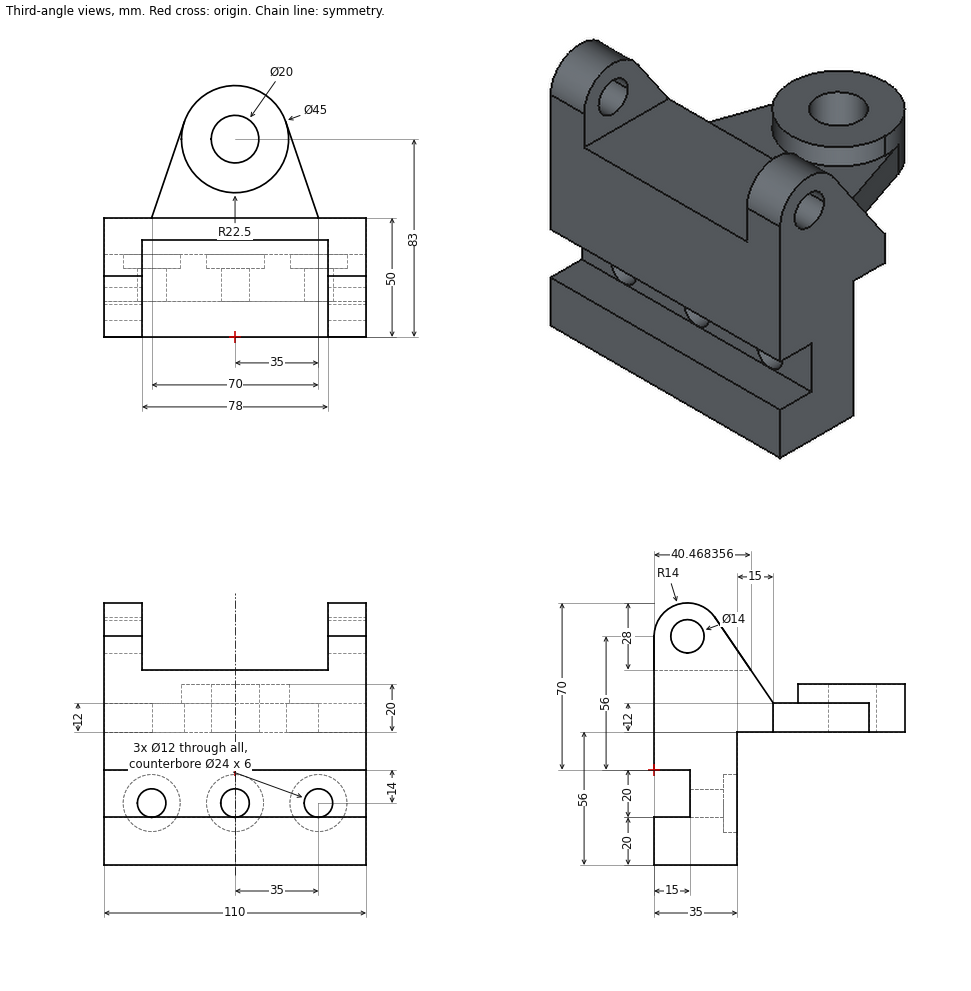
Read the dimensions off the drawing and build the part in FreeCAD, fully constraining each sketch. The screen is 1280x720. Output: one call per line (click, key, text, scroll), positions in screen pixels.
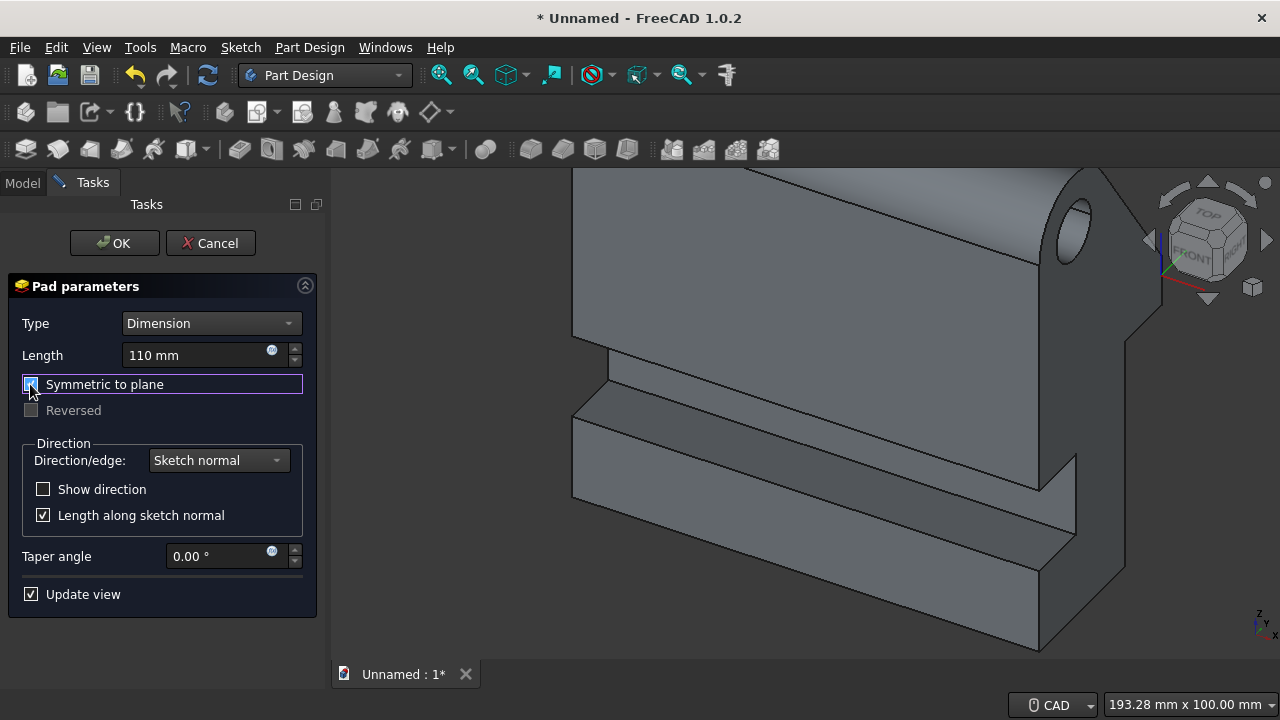
click(115, 243)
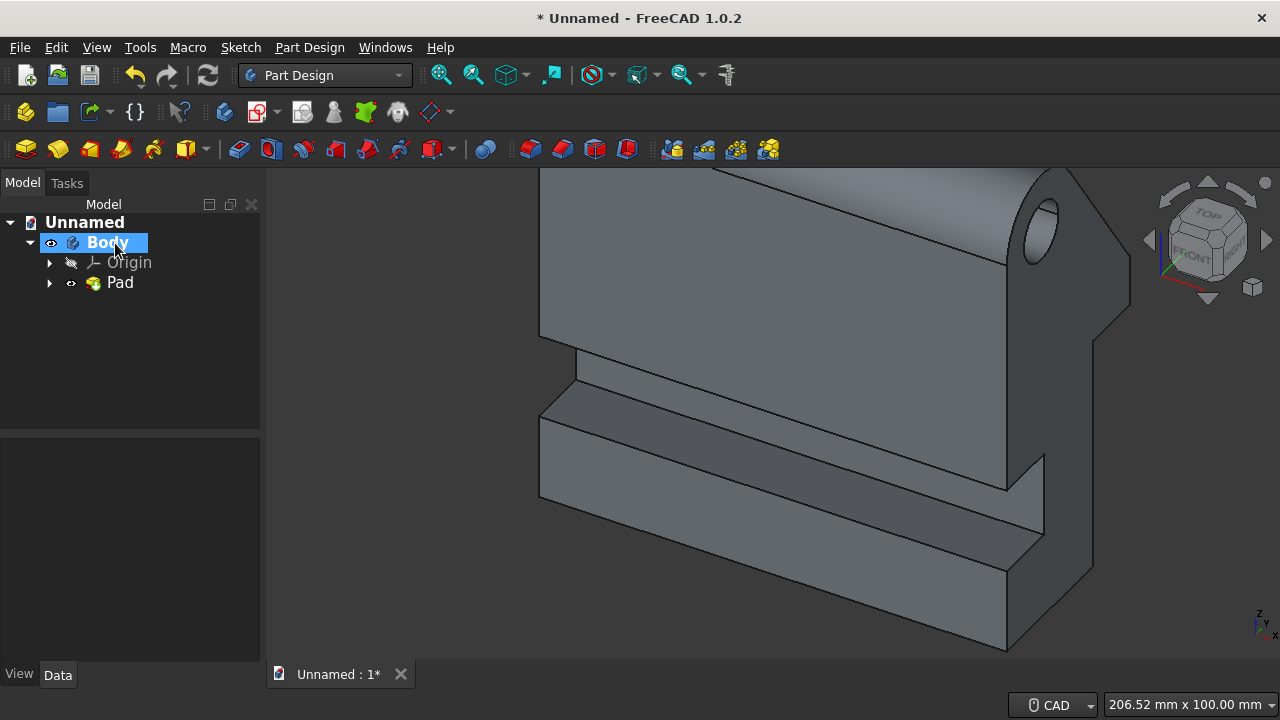
click(442, 76)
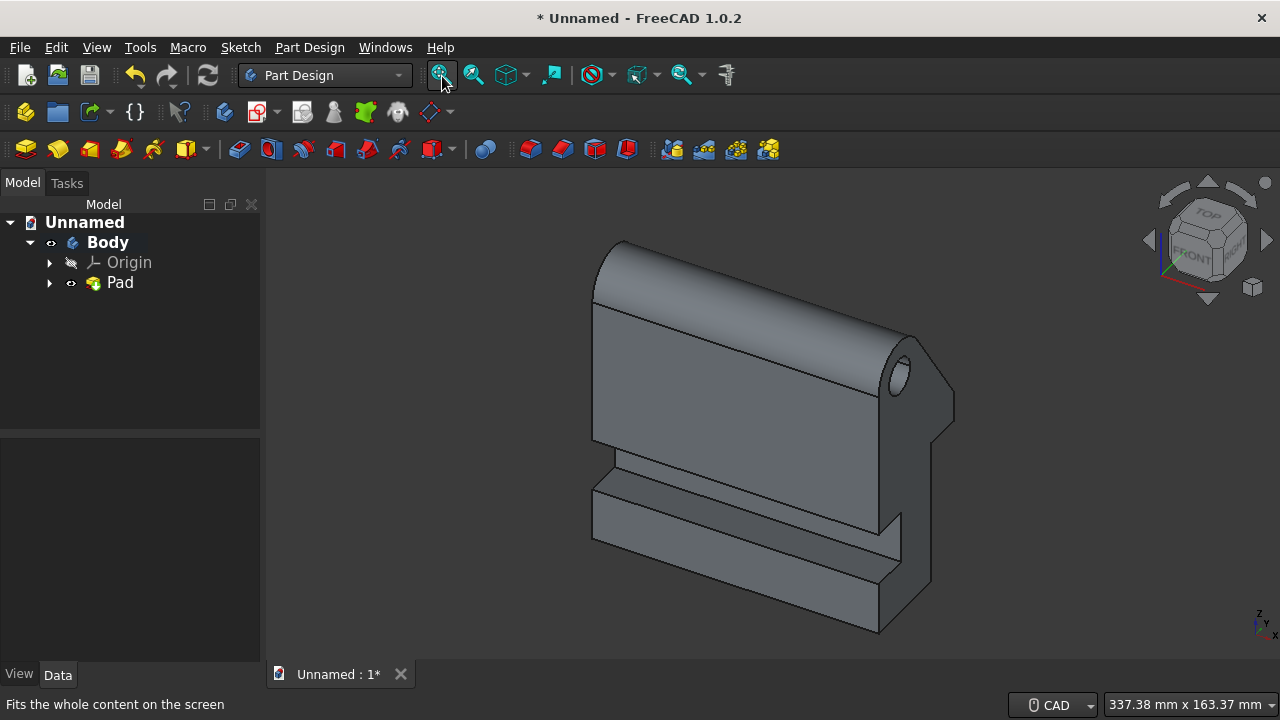
click(258, 112)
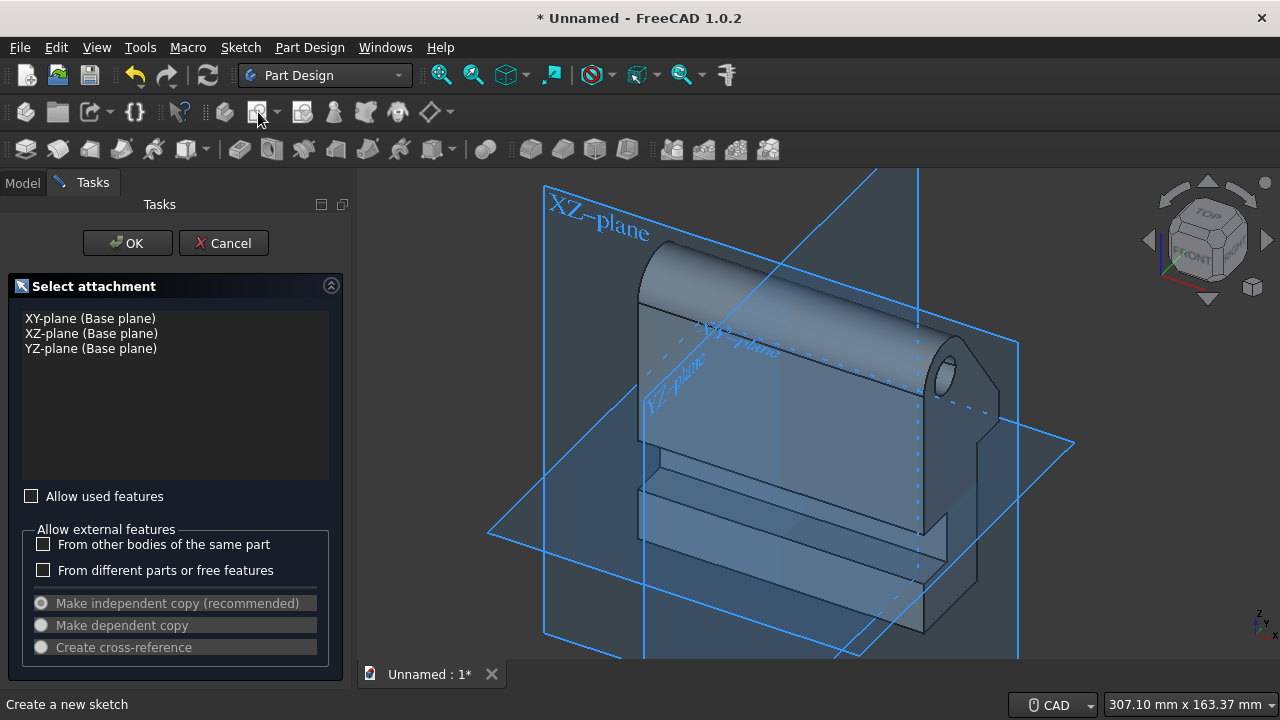
click(82, 348)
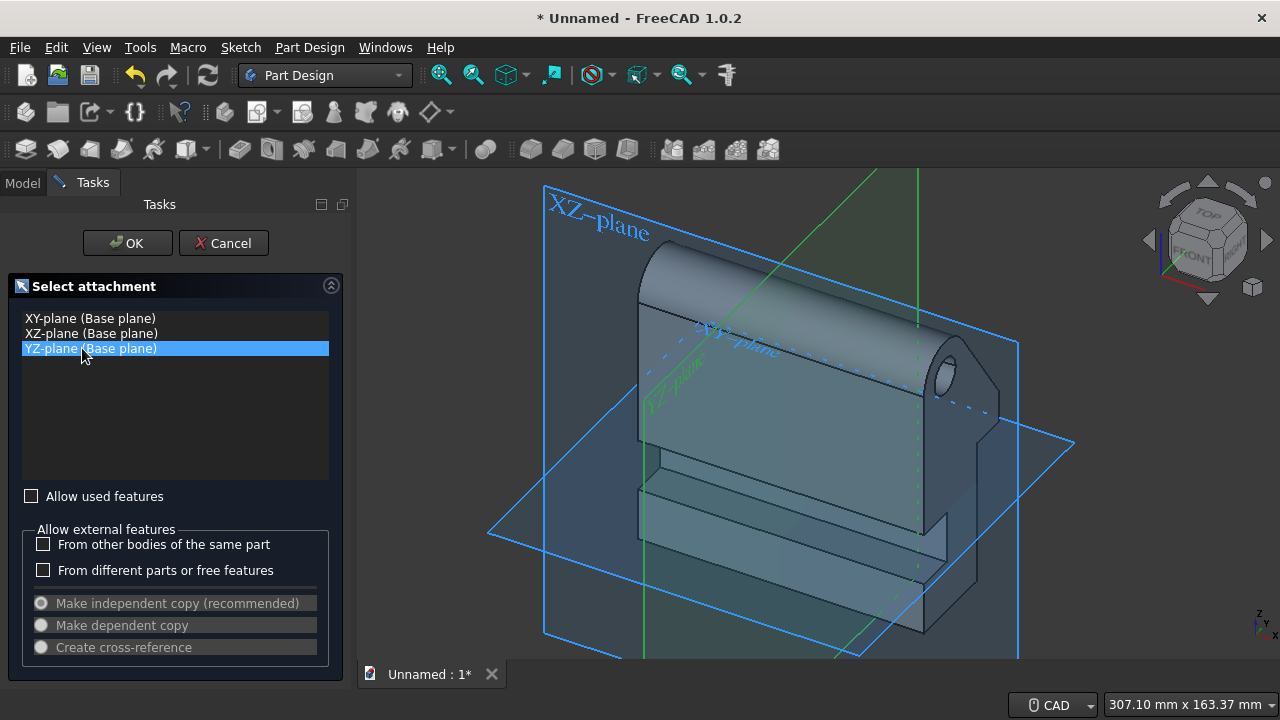
click(128, 243)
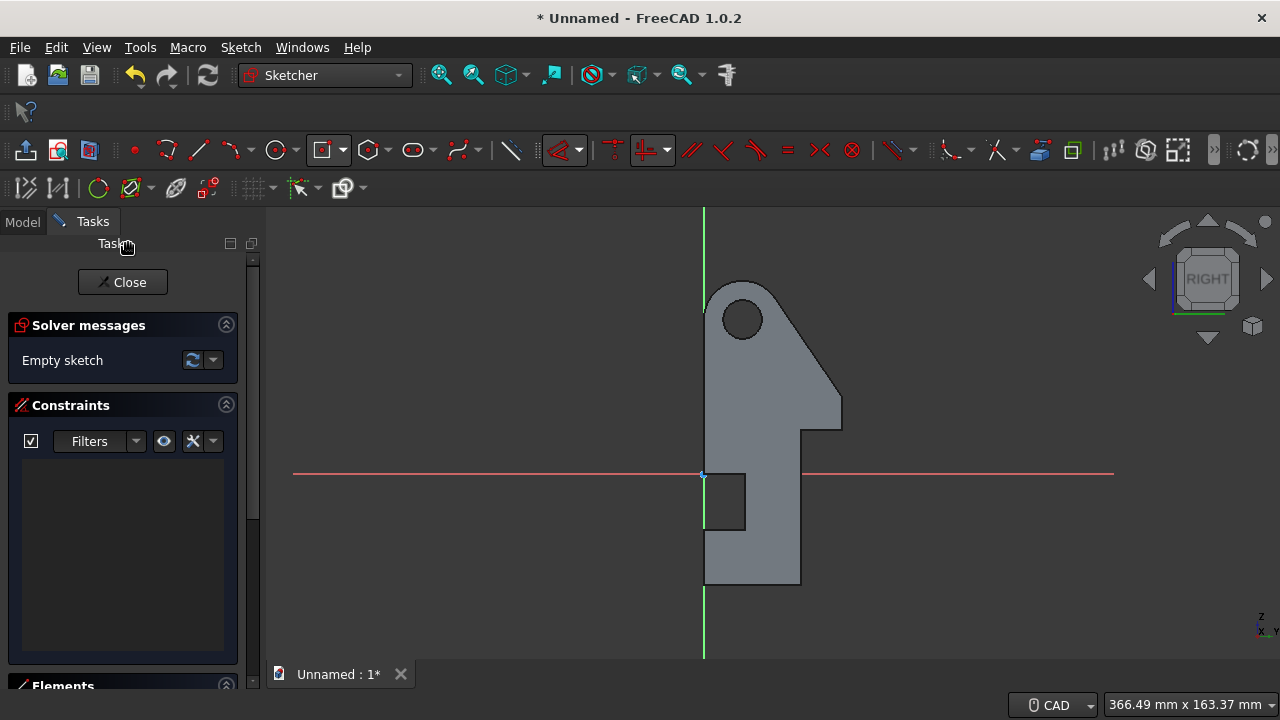
click(90, 150)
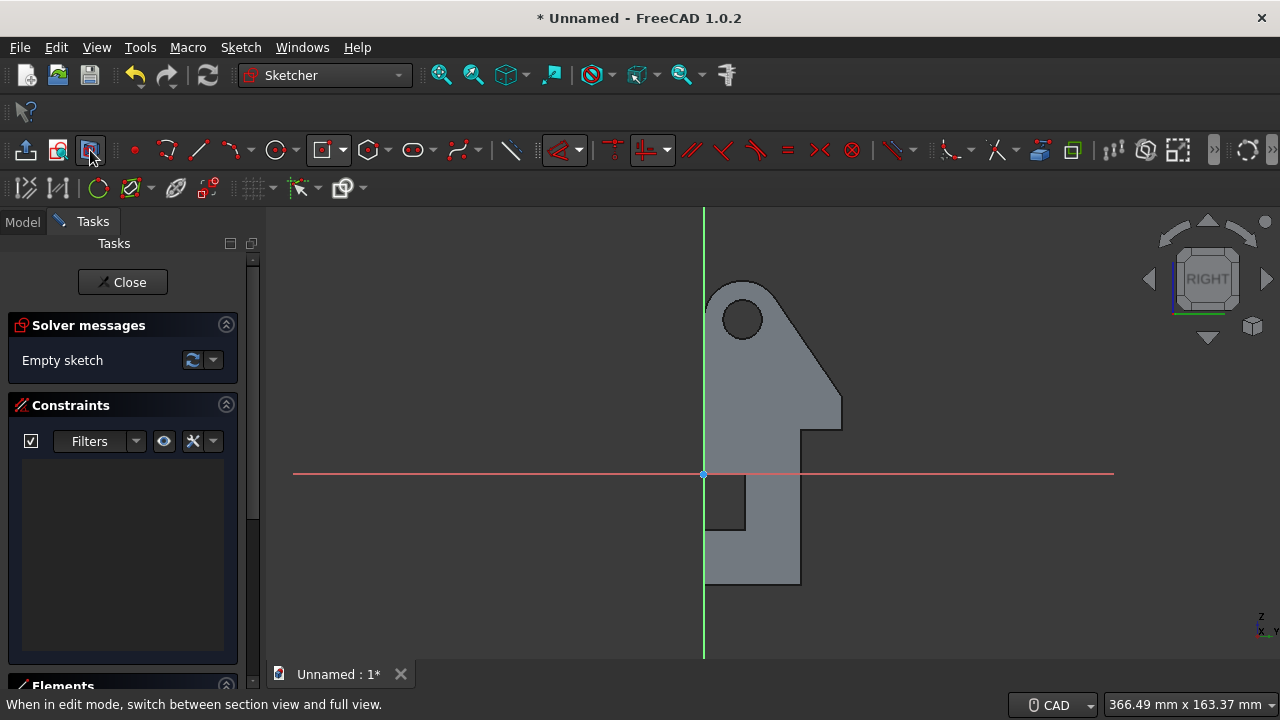
scroll(872, 265, up, 2)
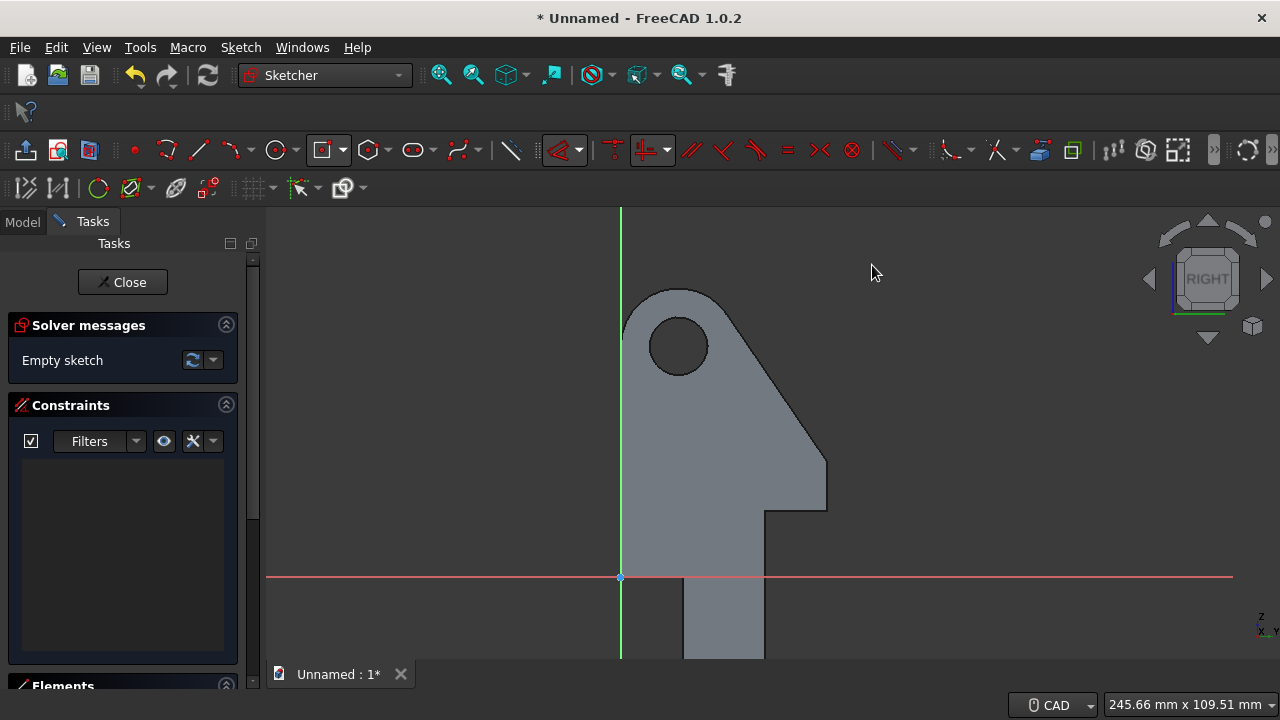
key(g)
key(r)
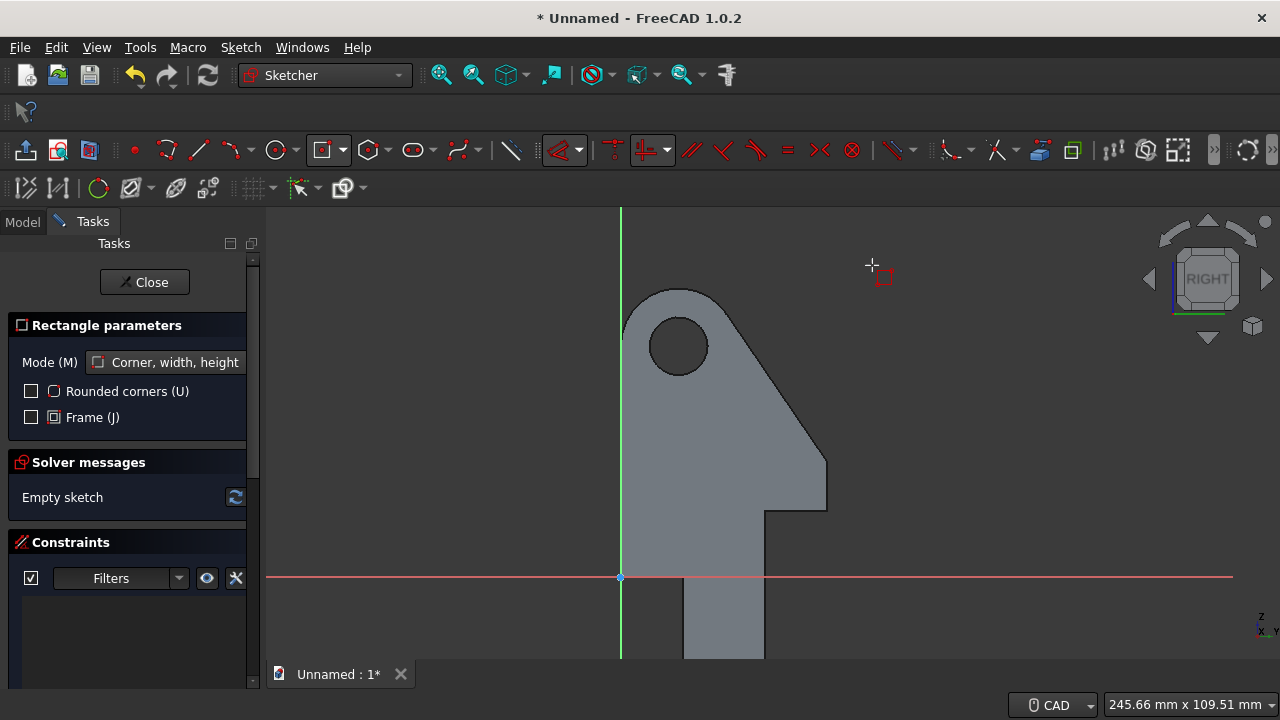
click(621, 288)
click(788, 404)
key(Escape)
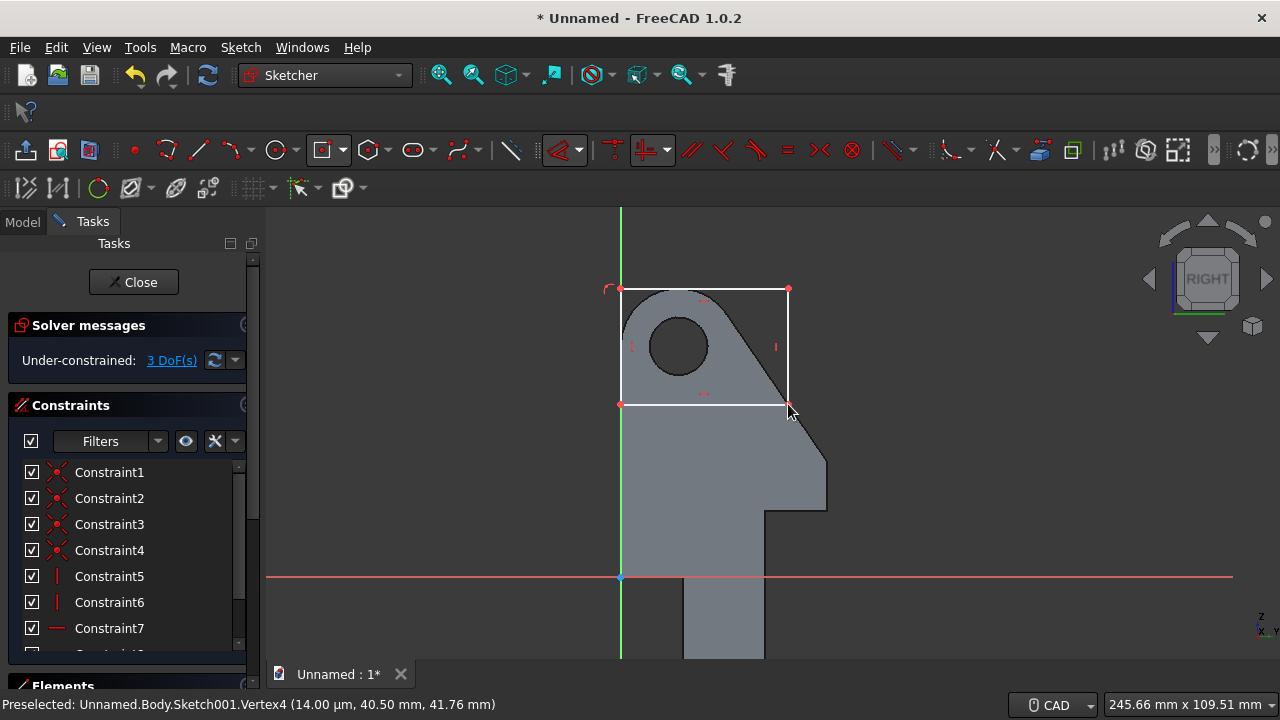
click(621, 324)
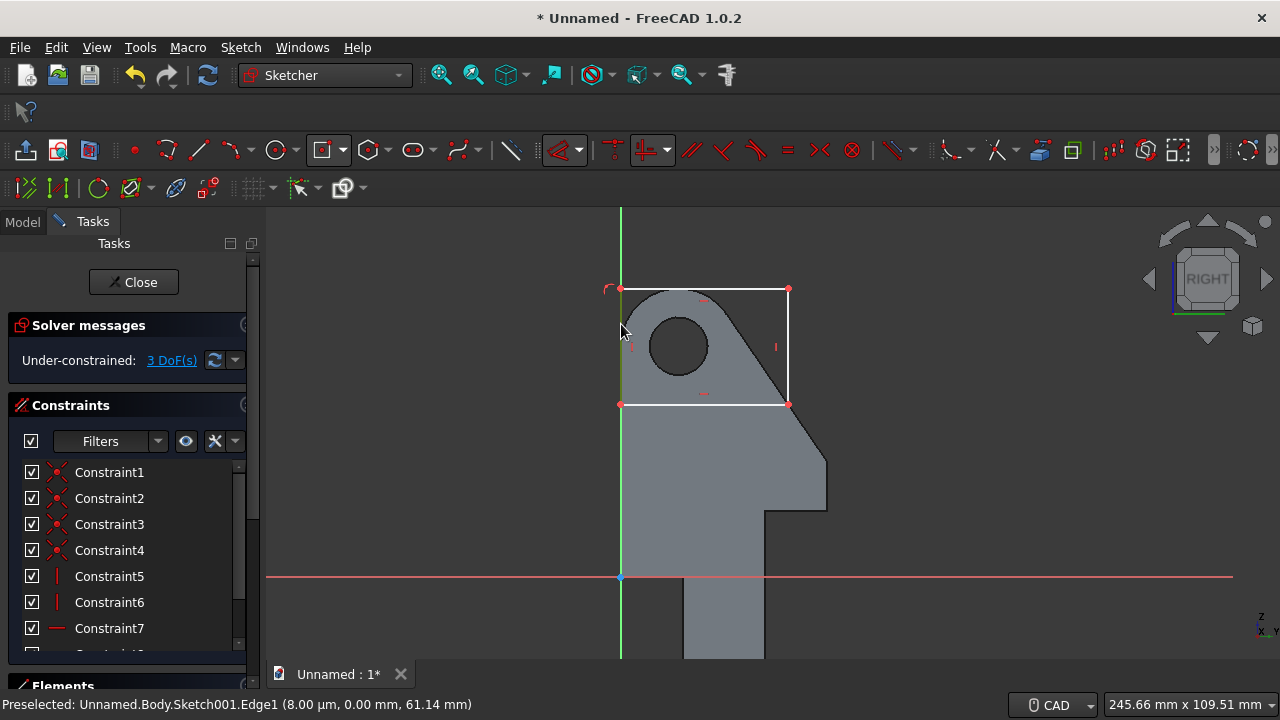
click(582, 150)